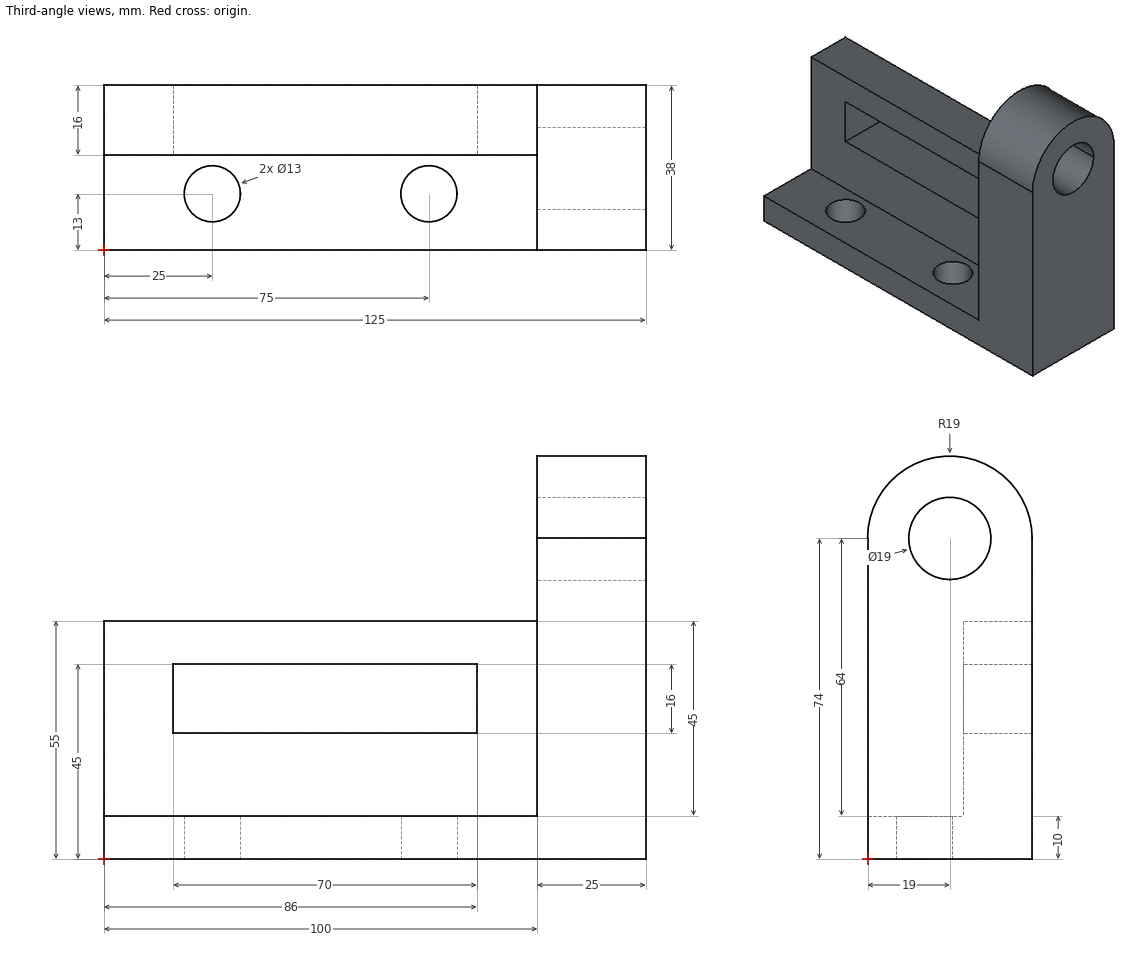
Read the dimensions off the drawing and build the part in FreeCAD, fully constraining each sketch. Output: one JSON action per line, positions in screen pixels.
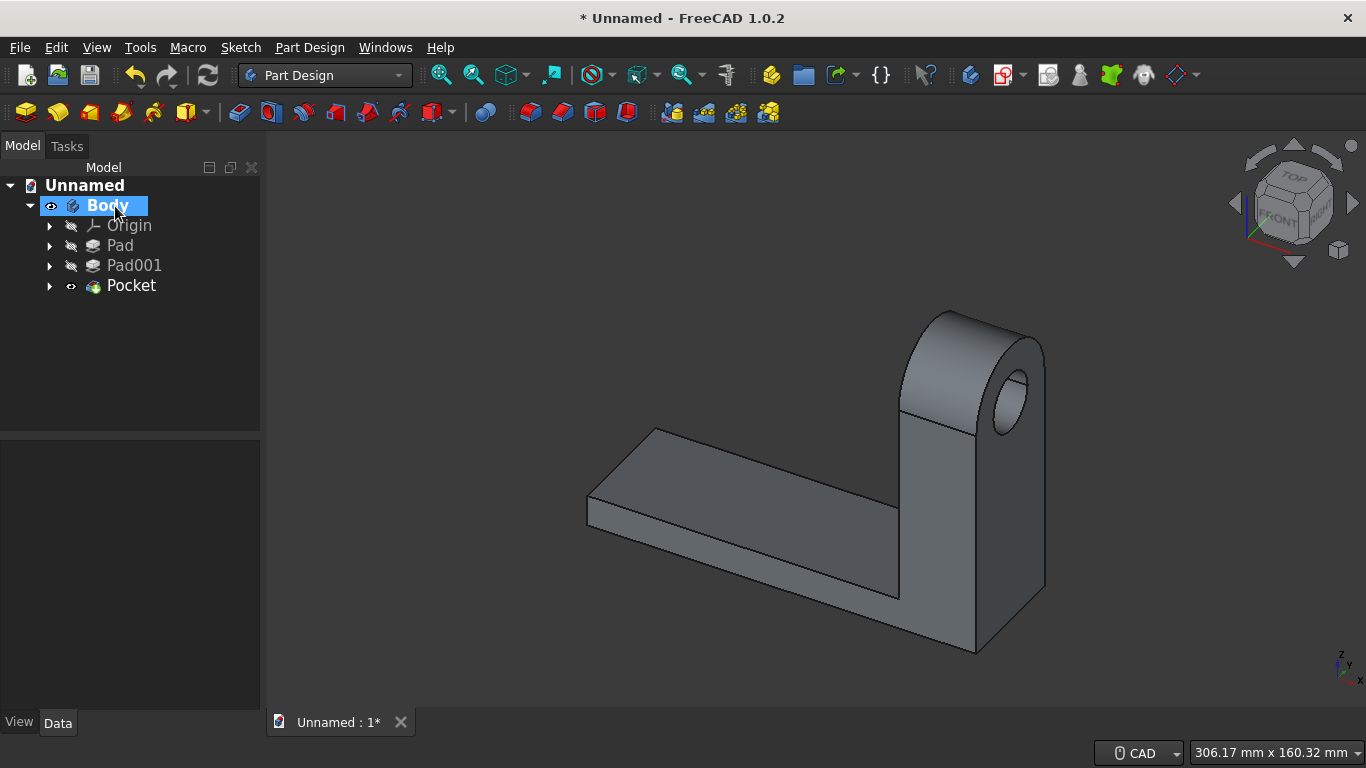
{"action": "key", "text": "4"}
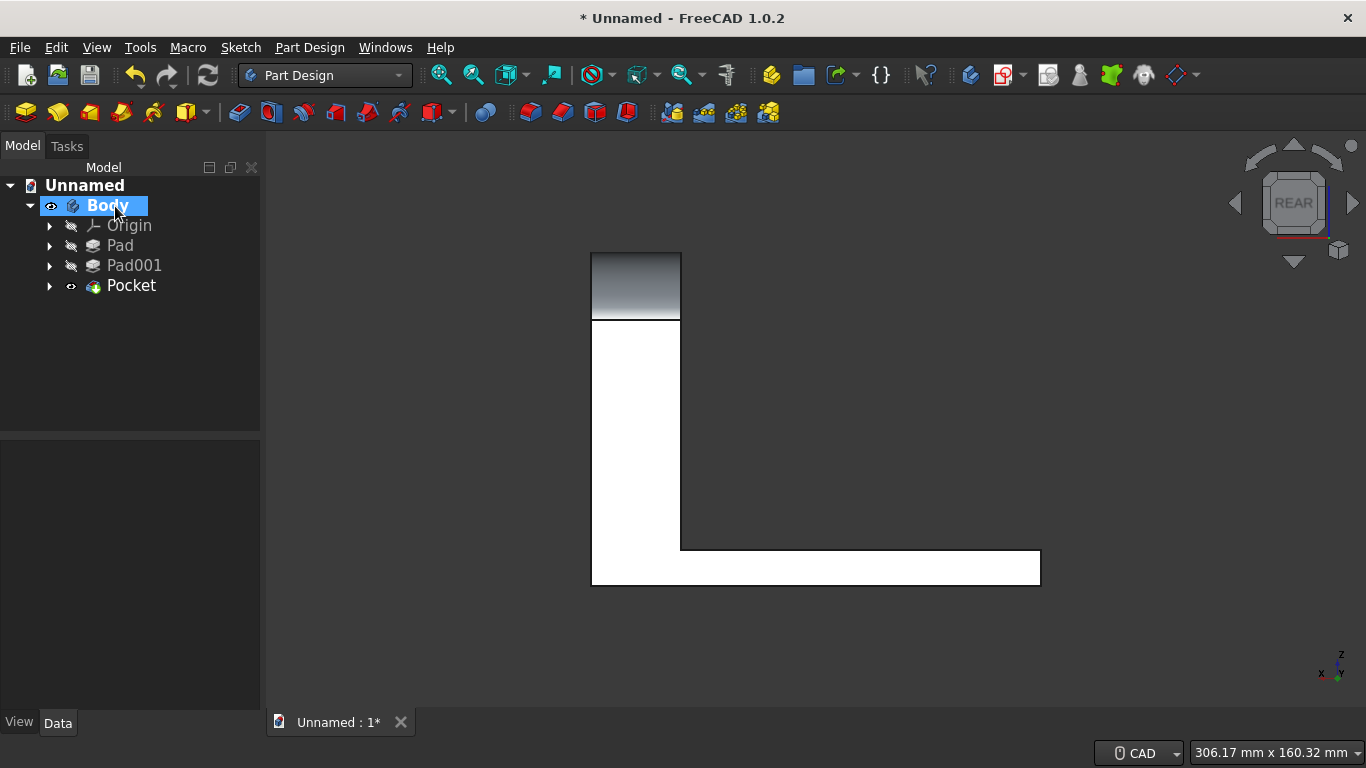
{"action": "left_click", "coordinate": [624, 376]}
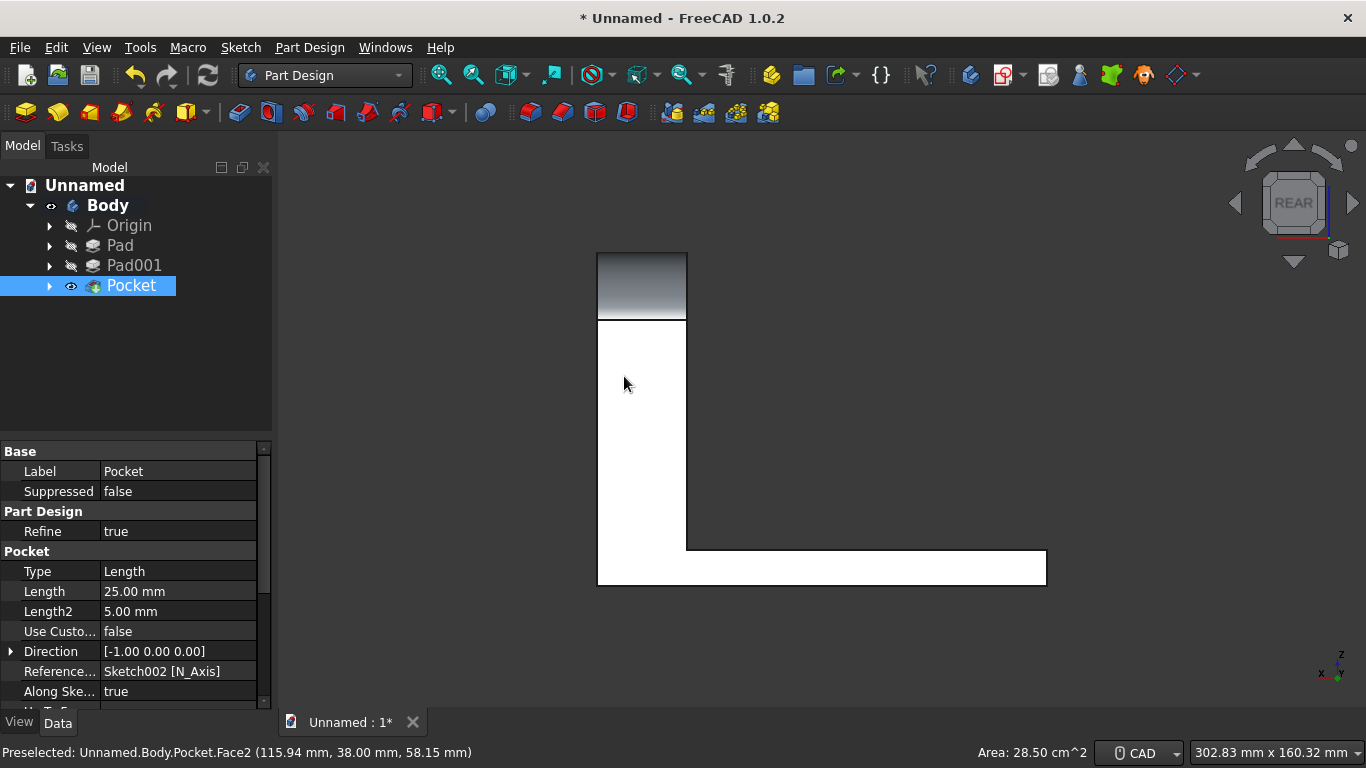
{"action": "left_click", "coordinate": [1004, 76]}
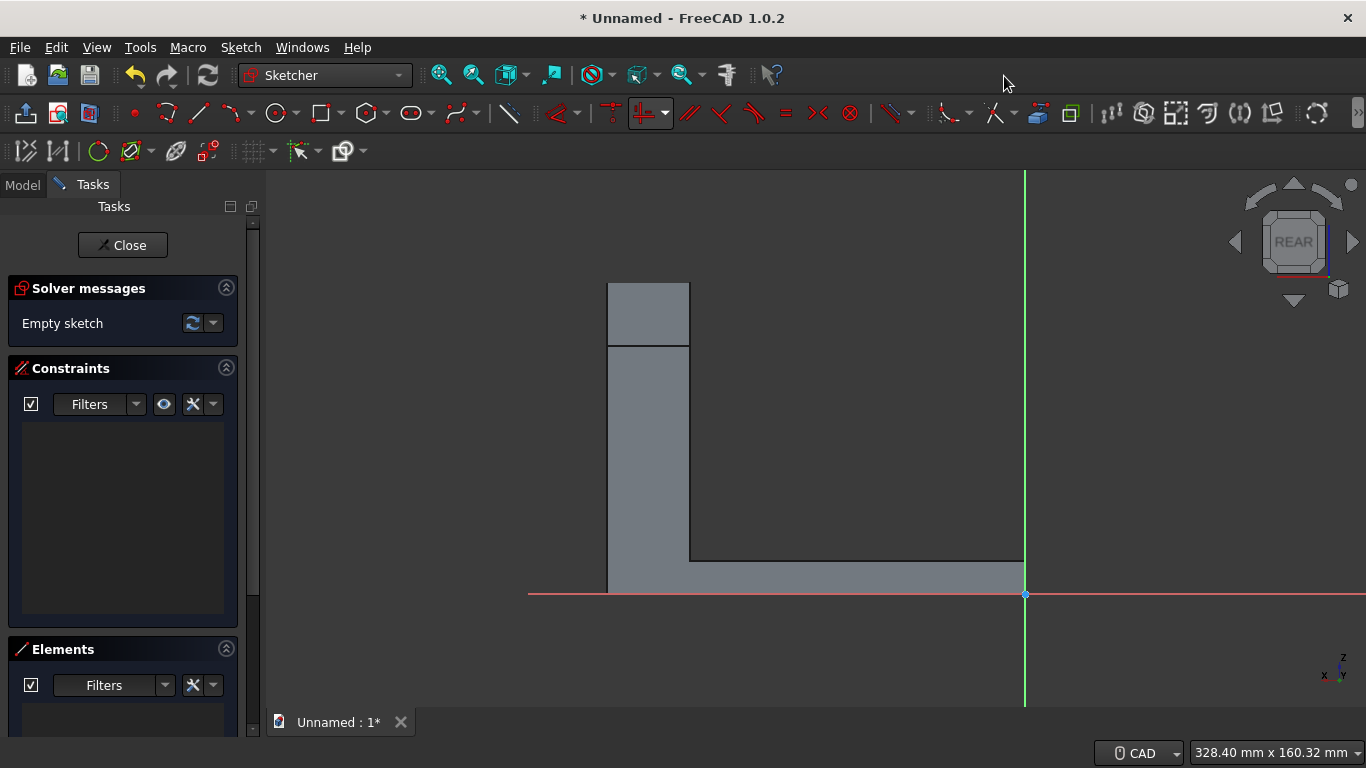
{"action": "scroll", "coordinate": [992, 579], "scroll_direction": "up", "scroll_amount": 3}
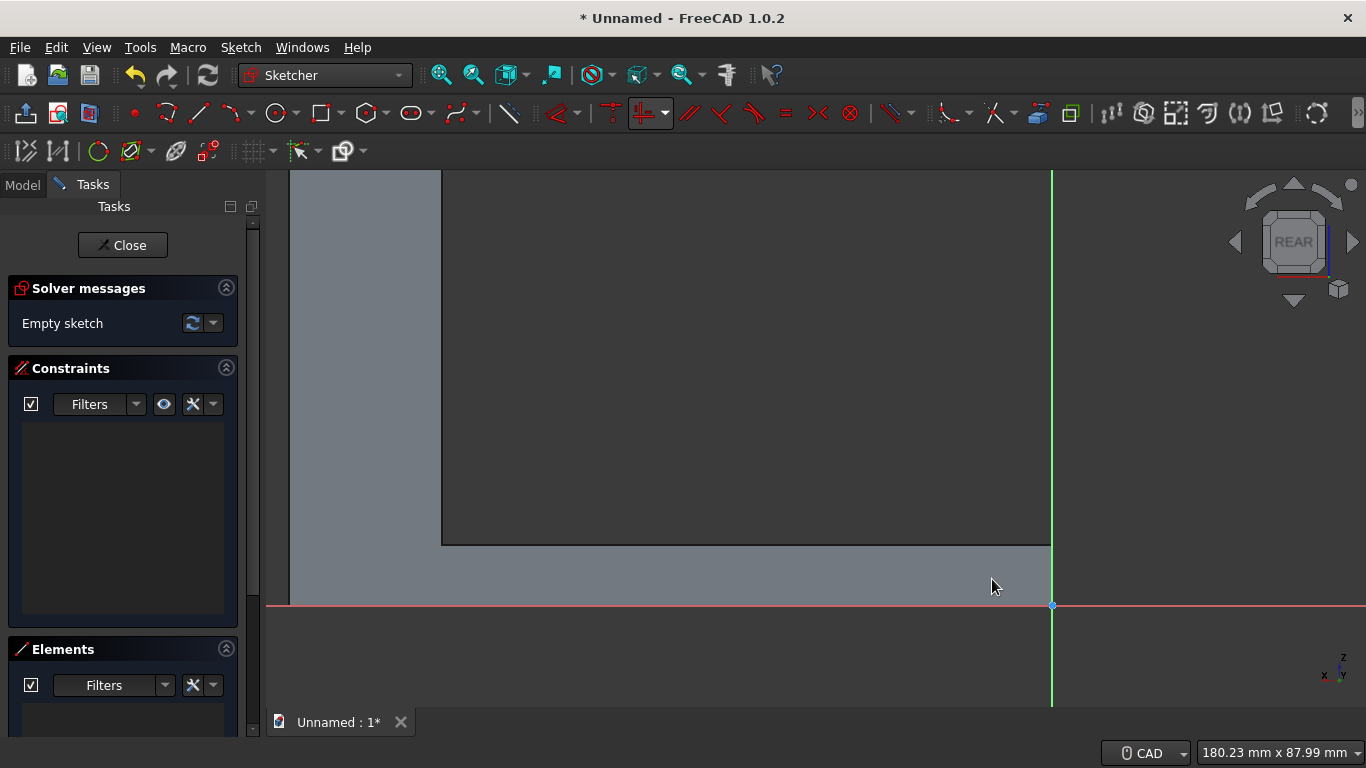
{"action": "left_click", "coordinate": [322, 114]}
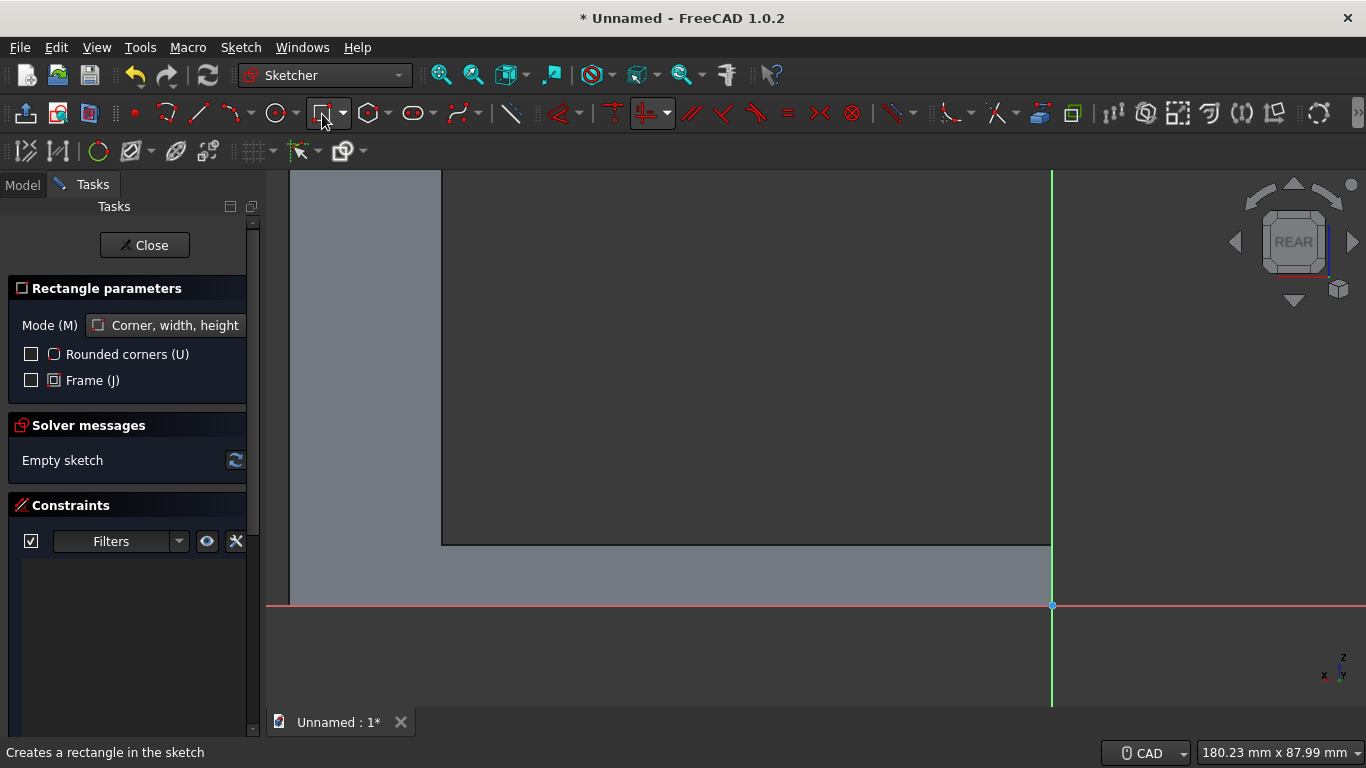
{"action": "left_click", "coordinate": [442, 270]}
{"action": "left_click", "coordinate": [1052, 545]}
{"action": "key", "text": "Escape"}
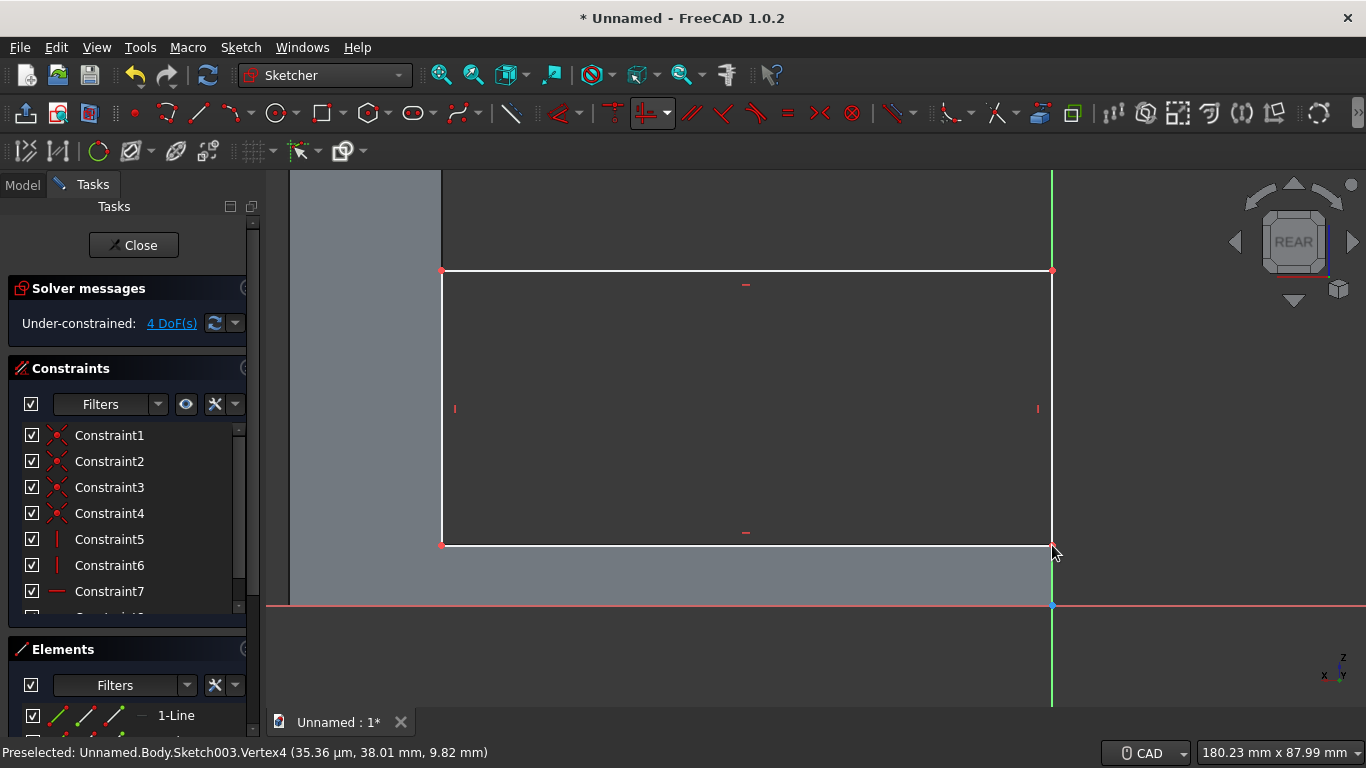
{"action": "left_click", "coordinate": [1052, 546]}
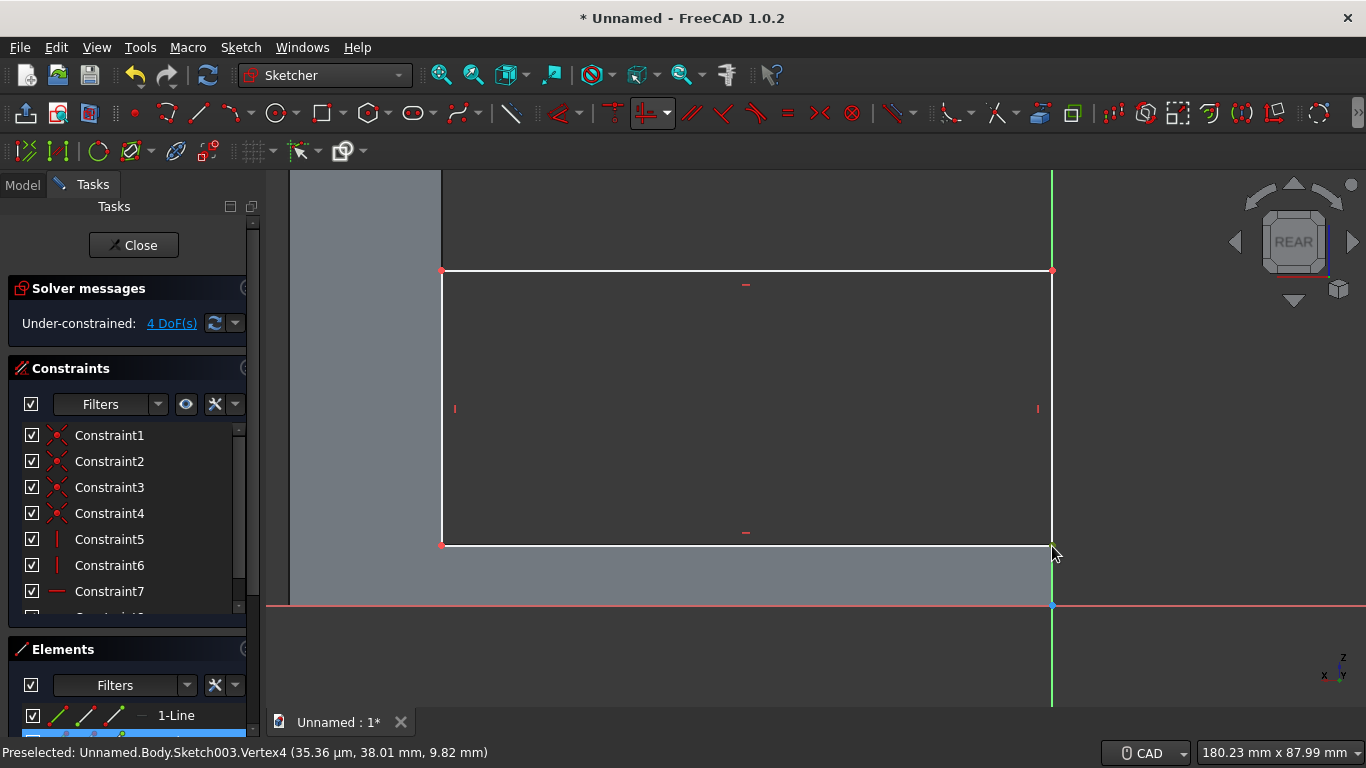
{"action": "left_click", "coordinate": [1052, 645]}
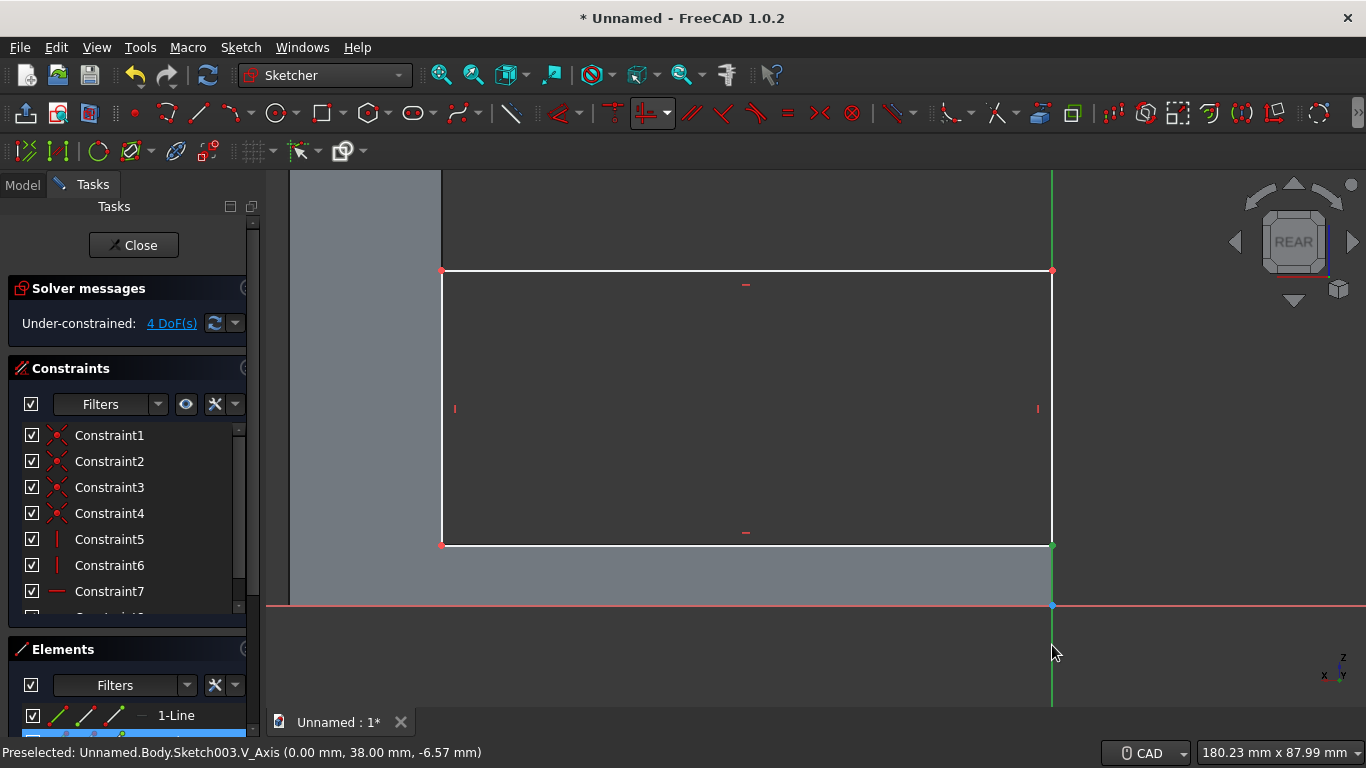
{"action": "left_click", "coordinate": [614, 114]}